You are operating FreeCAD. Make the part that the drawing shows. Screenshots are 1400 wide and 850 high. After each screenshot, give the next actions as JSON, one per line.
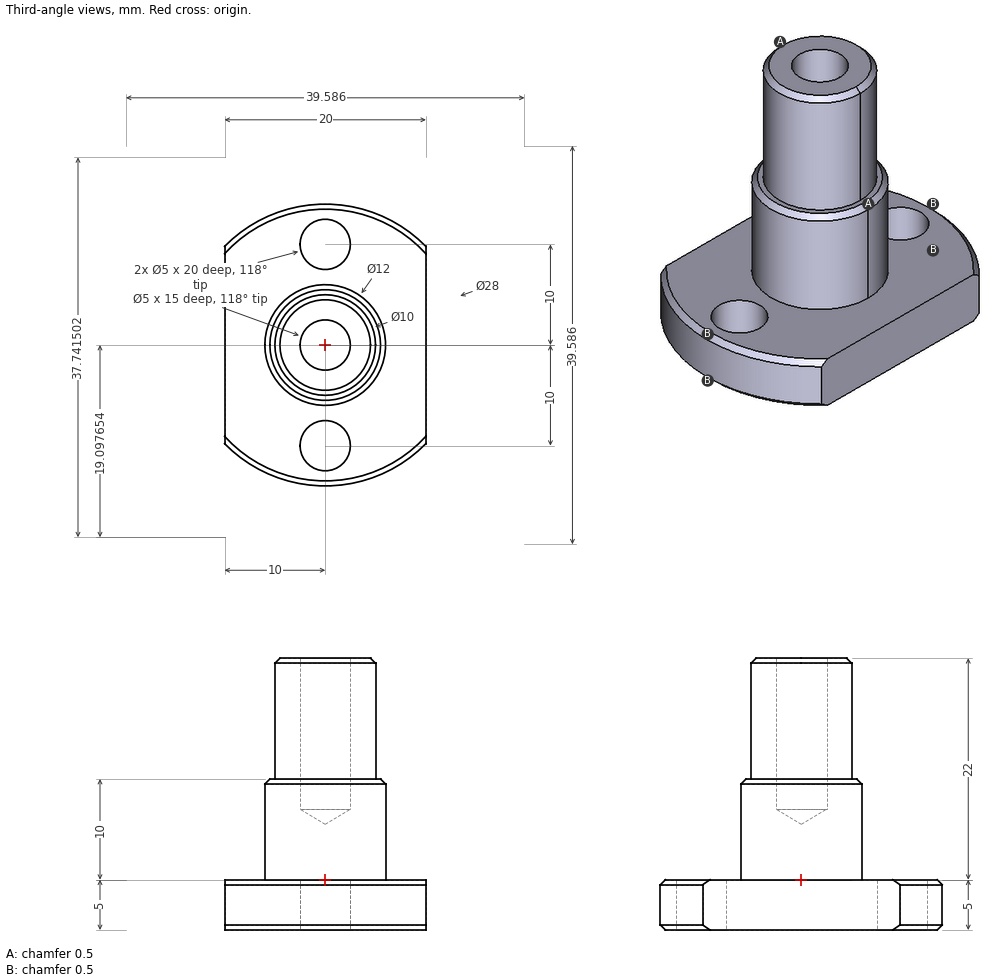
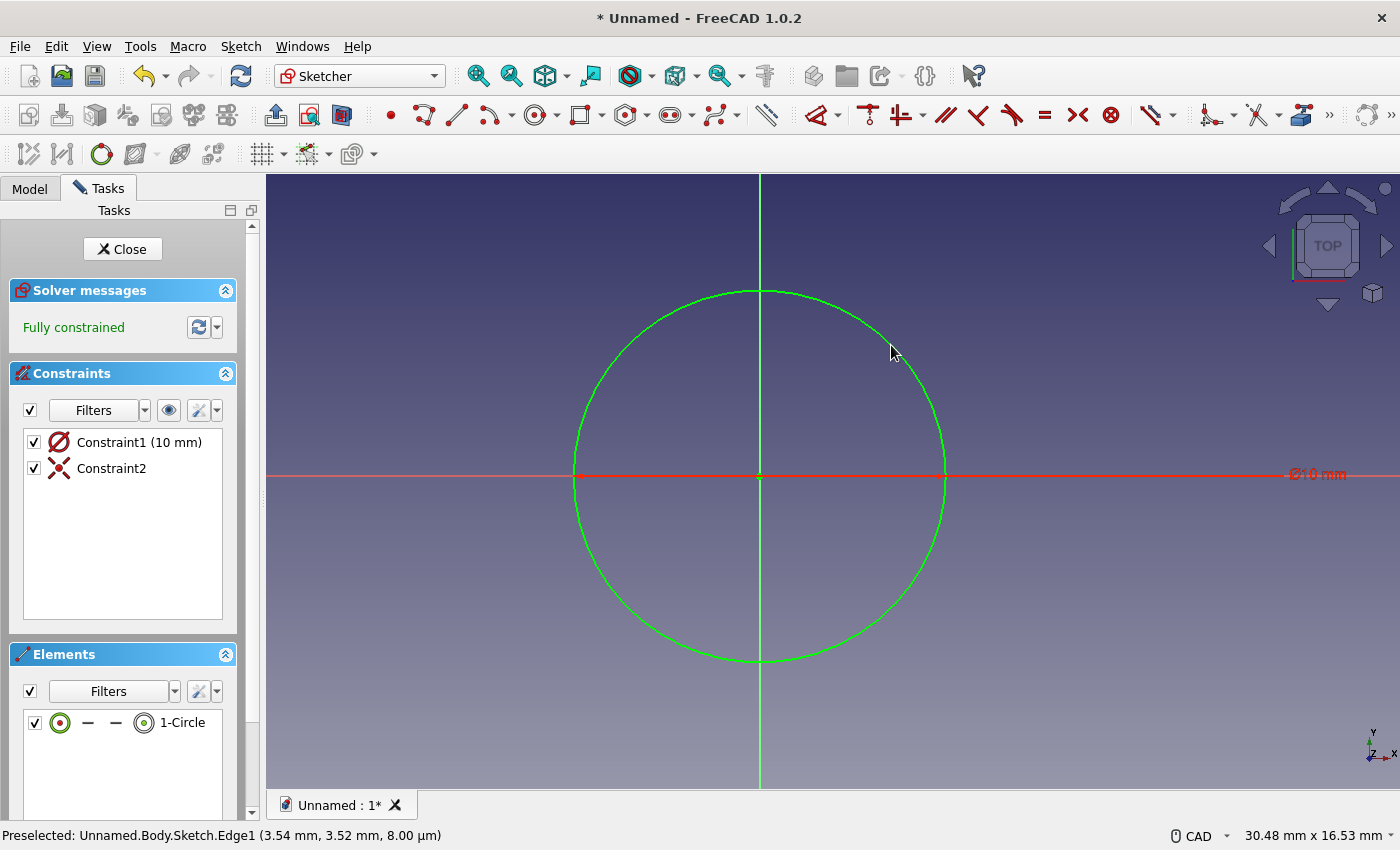
{"action": "left_click", "coordinate": [123, 249]}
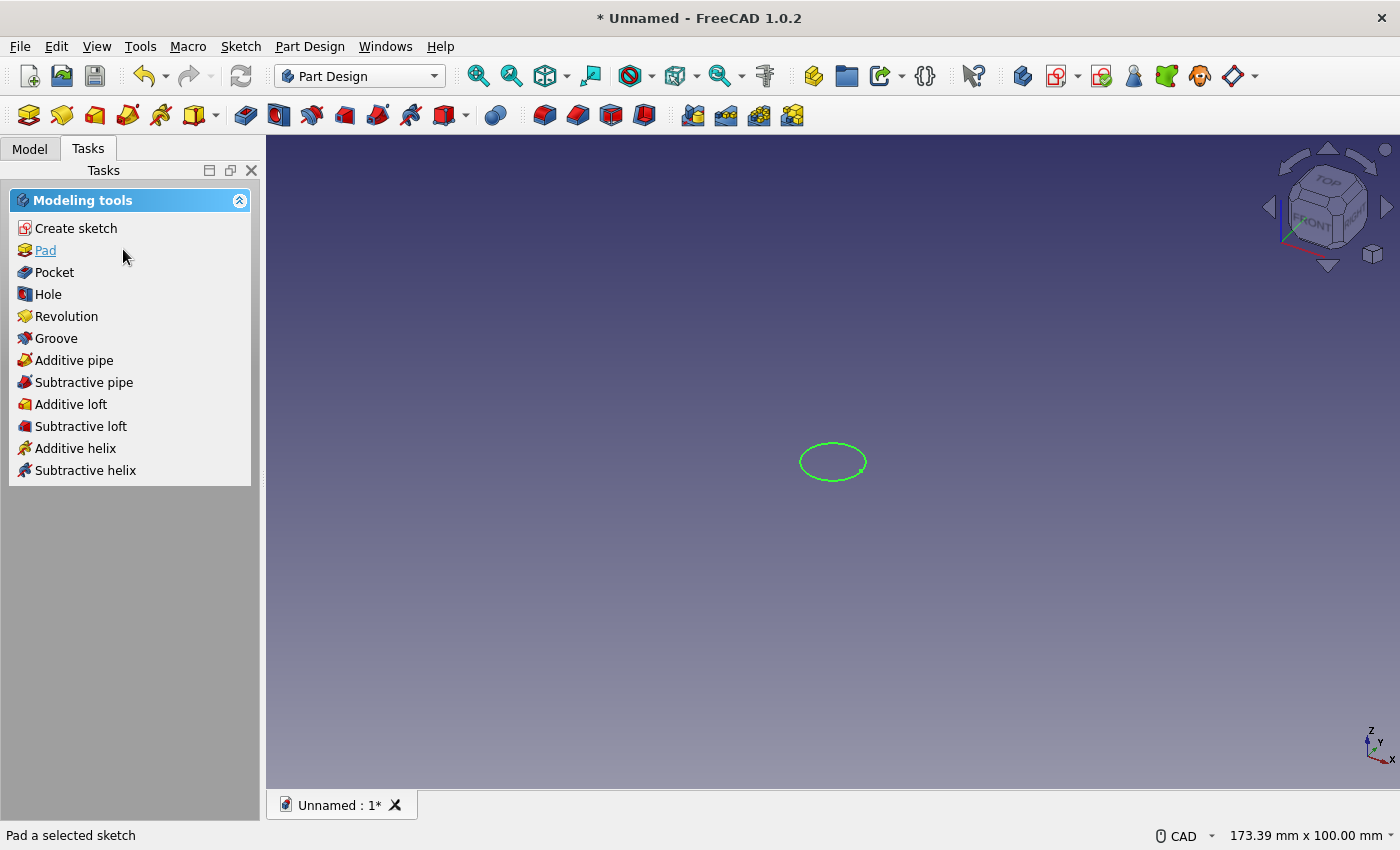
{"action": "left_click", "coordinate": [29, 116]}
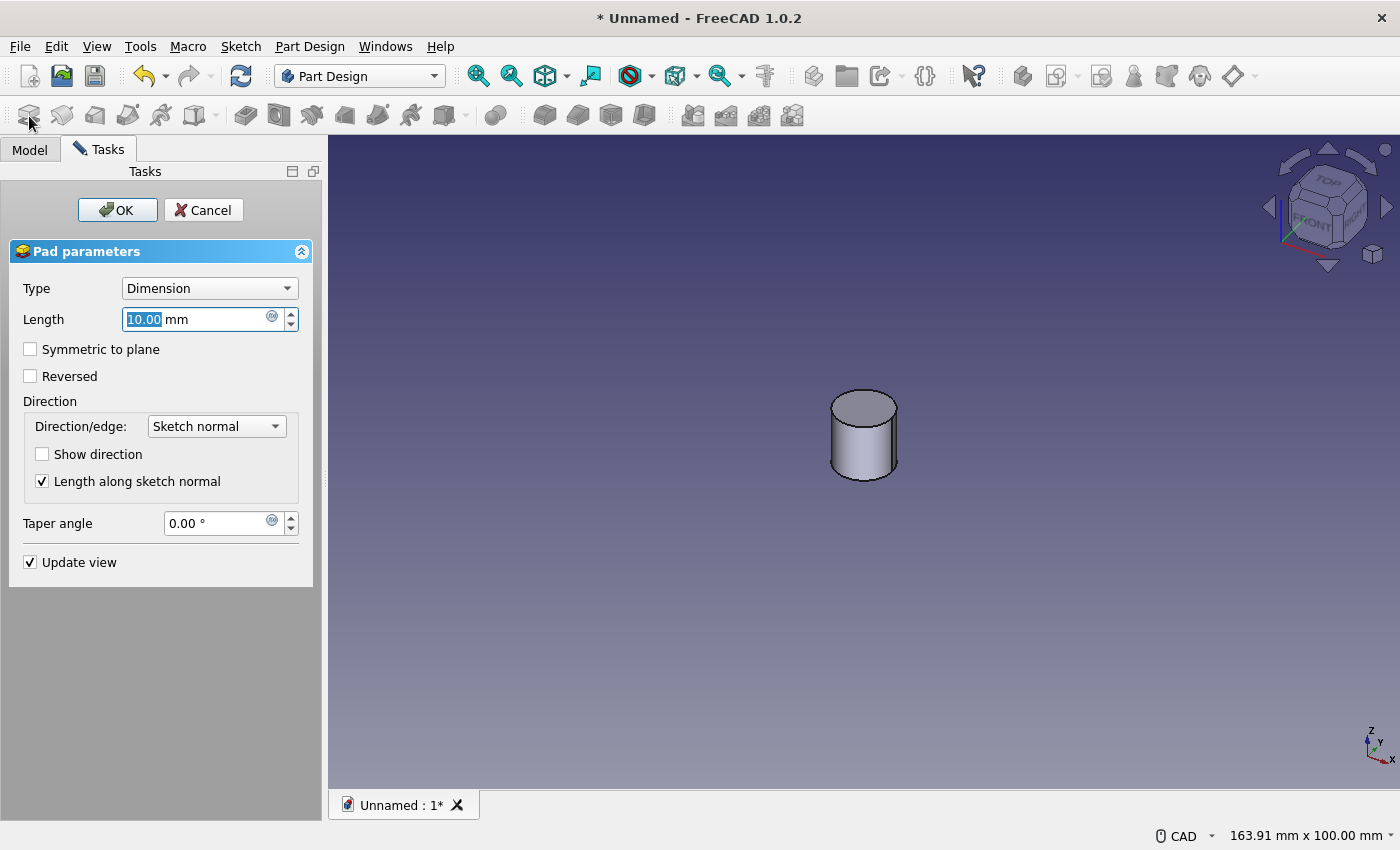
{"action": "type", "text": "22"}
{"action": "key", "text": "Tab"}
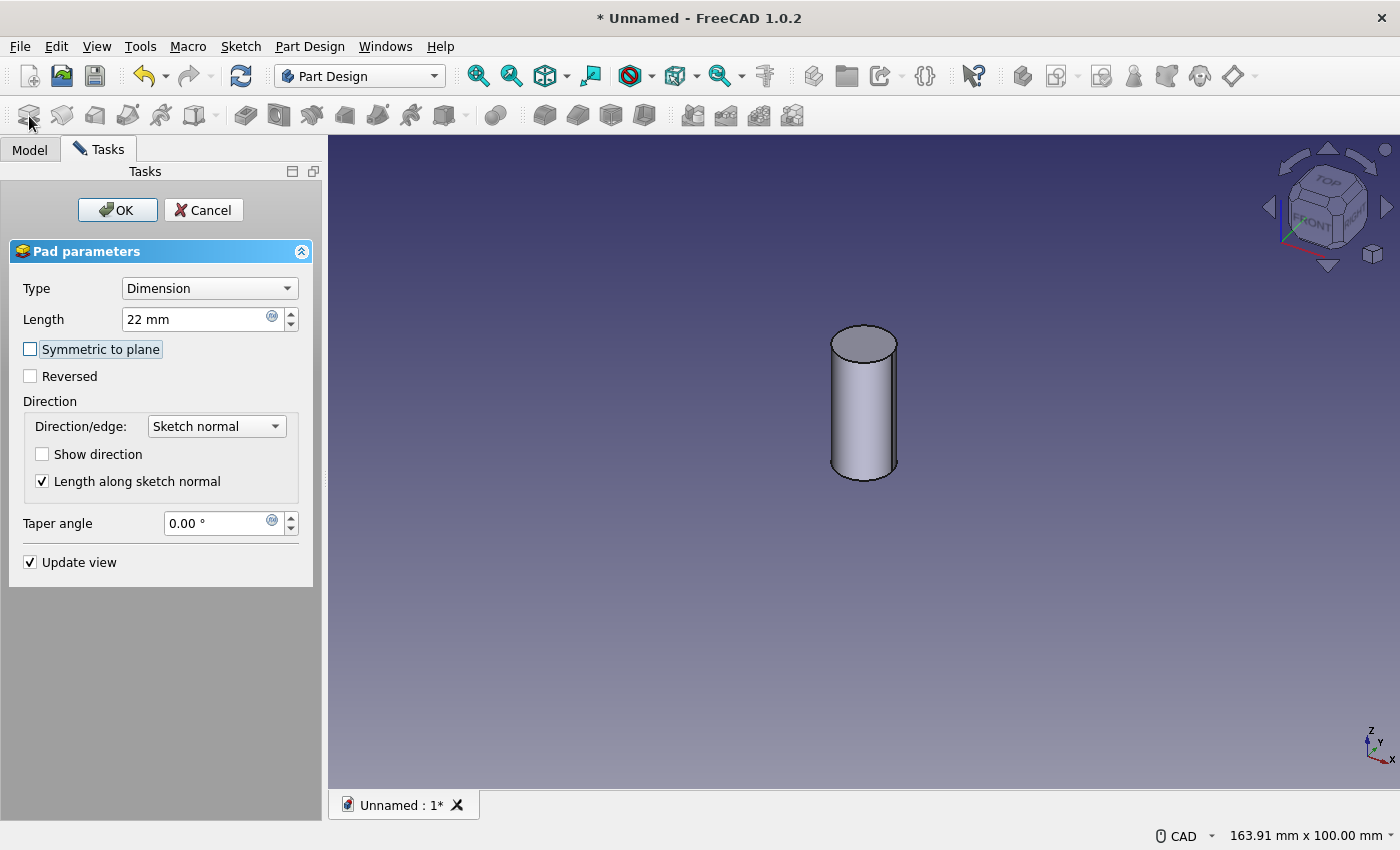
{"action": "left_click", "coordinate": [118, 210]}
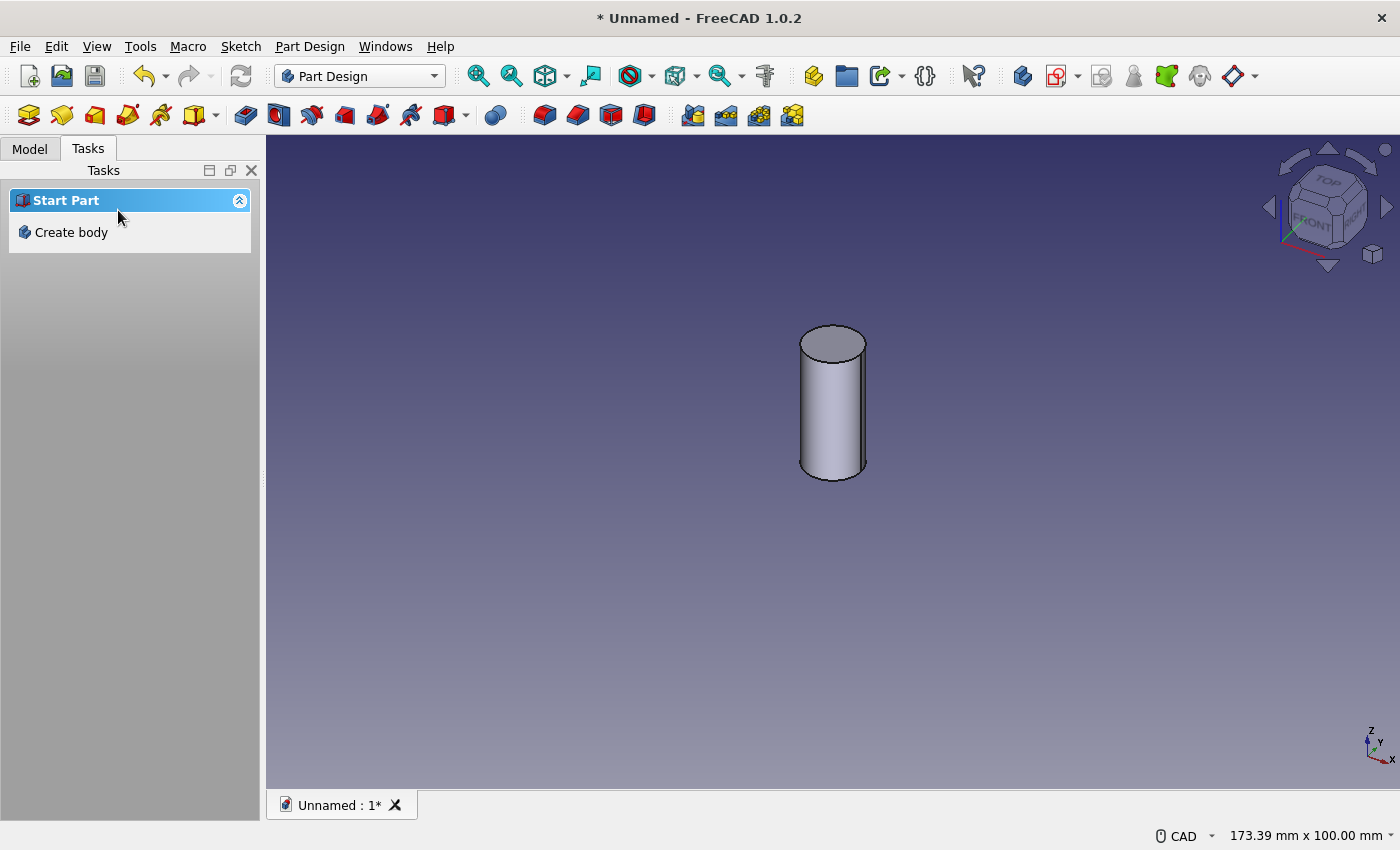
{"action": "left_click", "coordinate": [479, 76]}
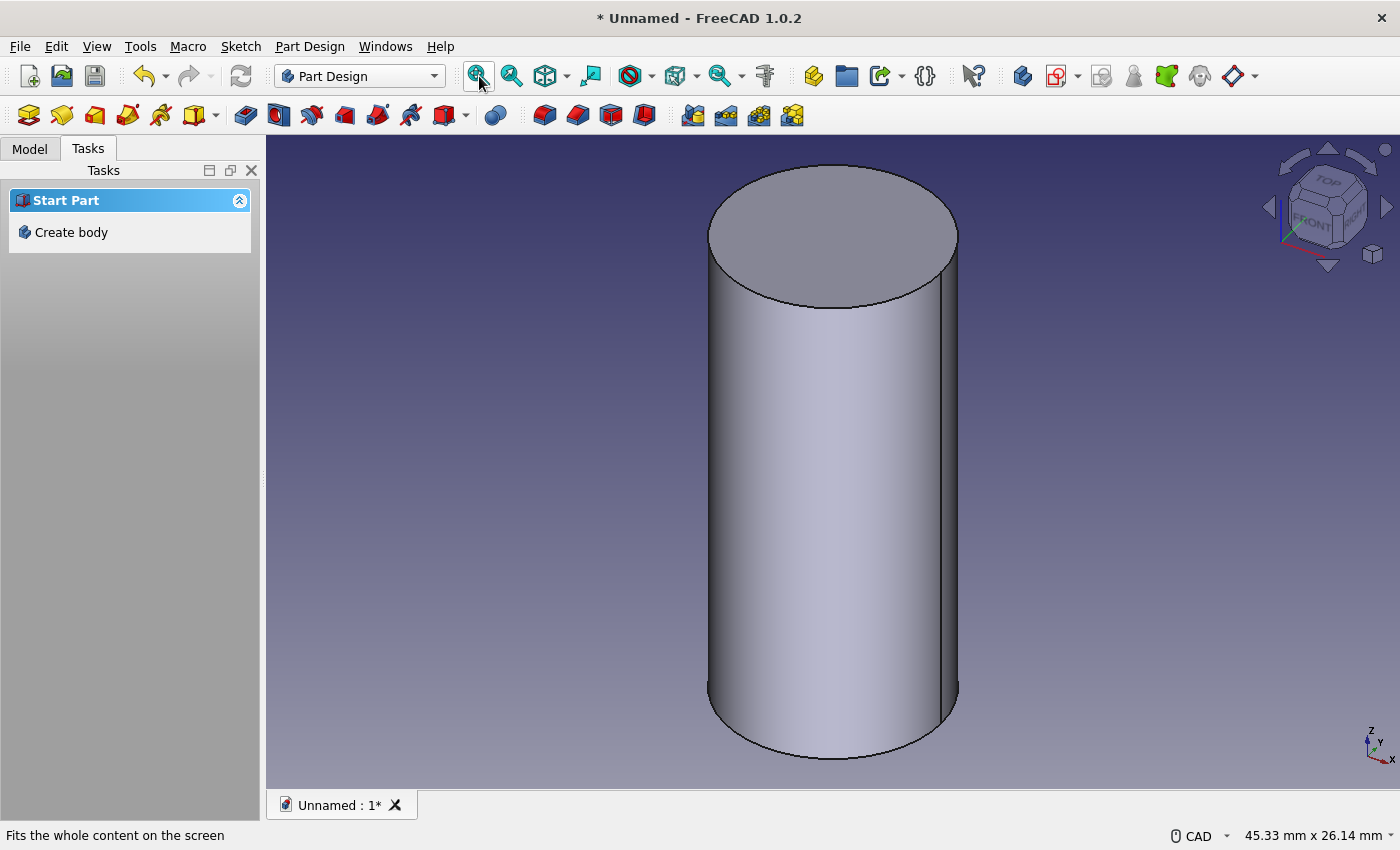
{"action": "left_click", "coordinate": [1056, 76]}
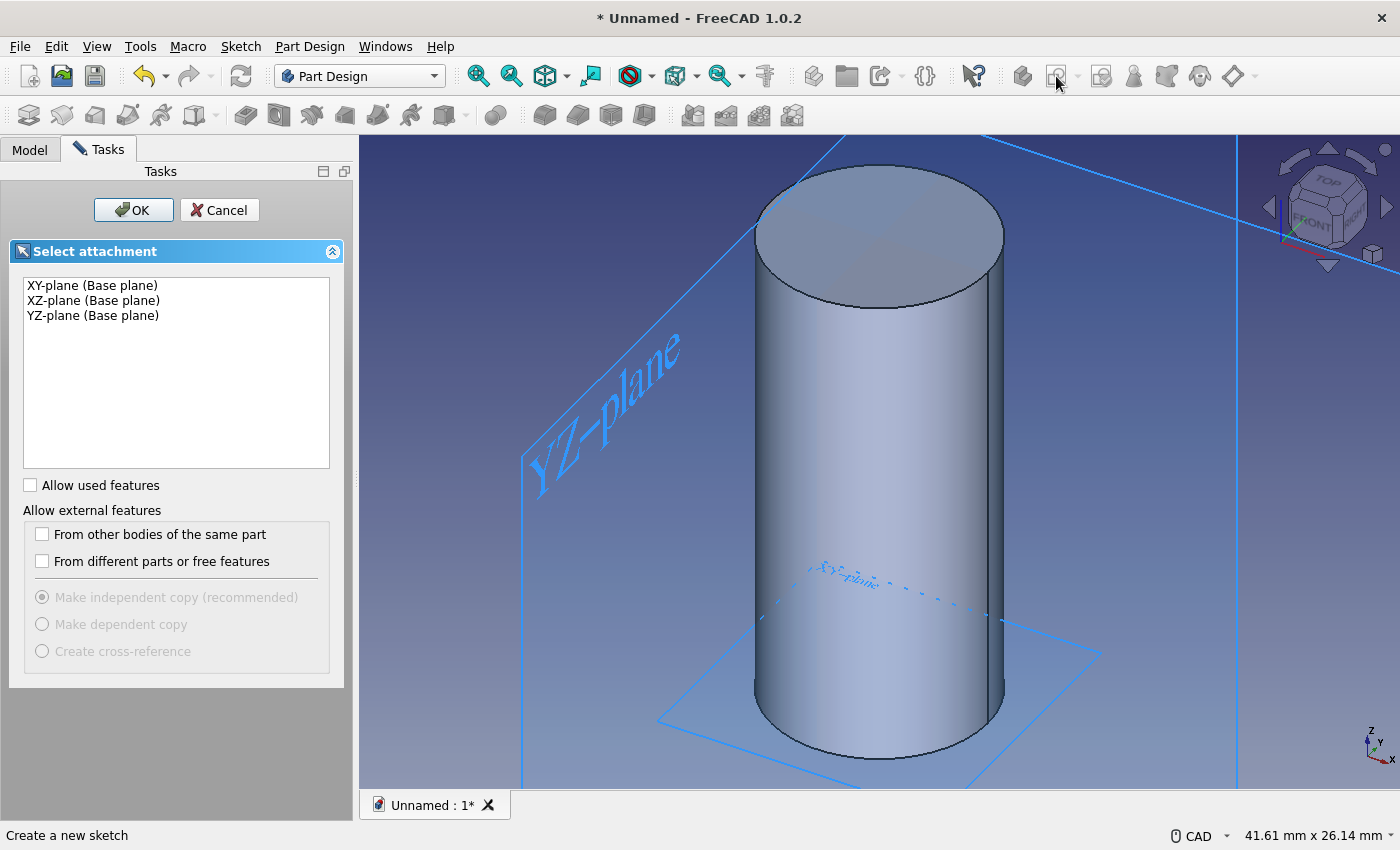
{"action": "left_click", "coordinate": [84, 286]}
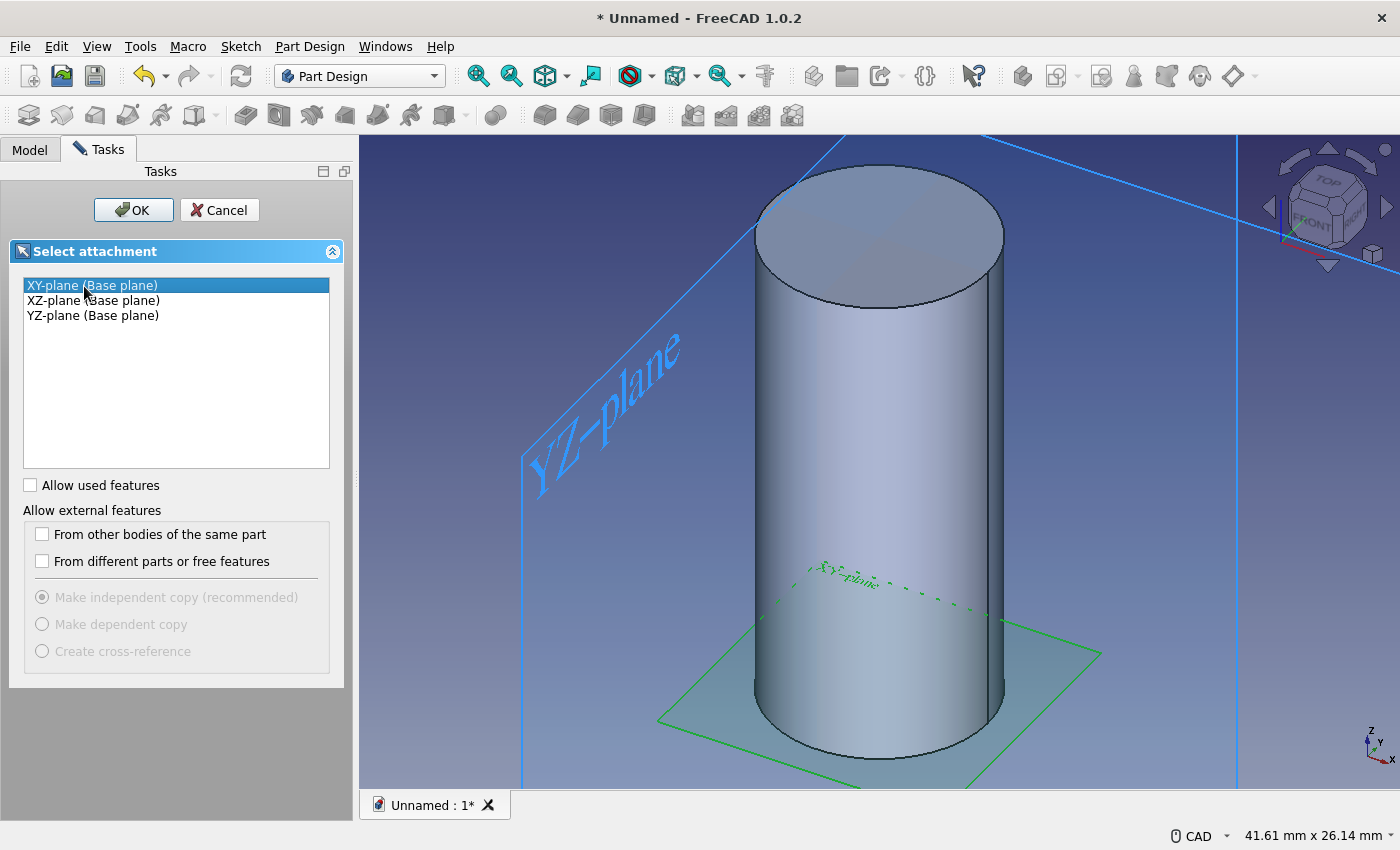
{"action": "left_click", "coordinate": [134, 210]}